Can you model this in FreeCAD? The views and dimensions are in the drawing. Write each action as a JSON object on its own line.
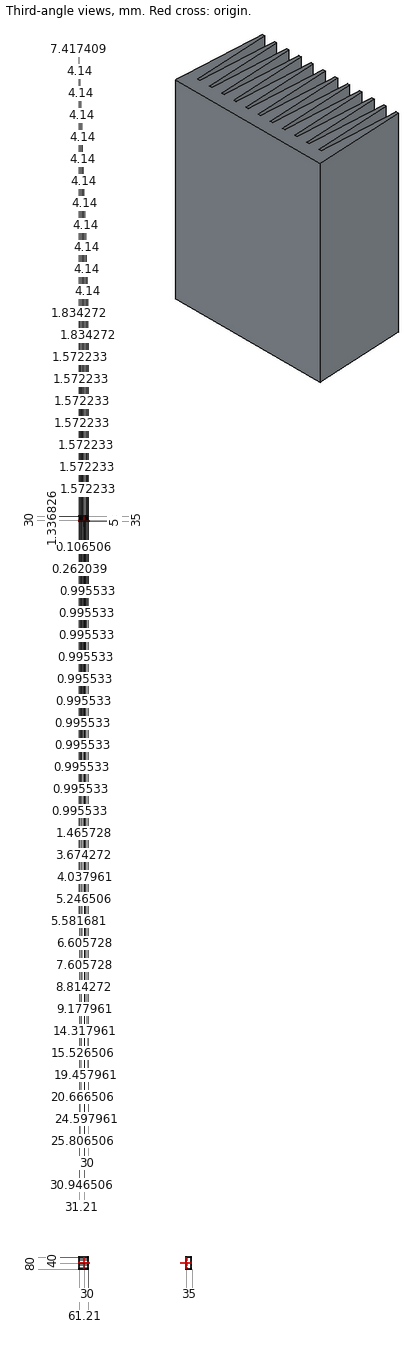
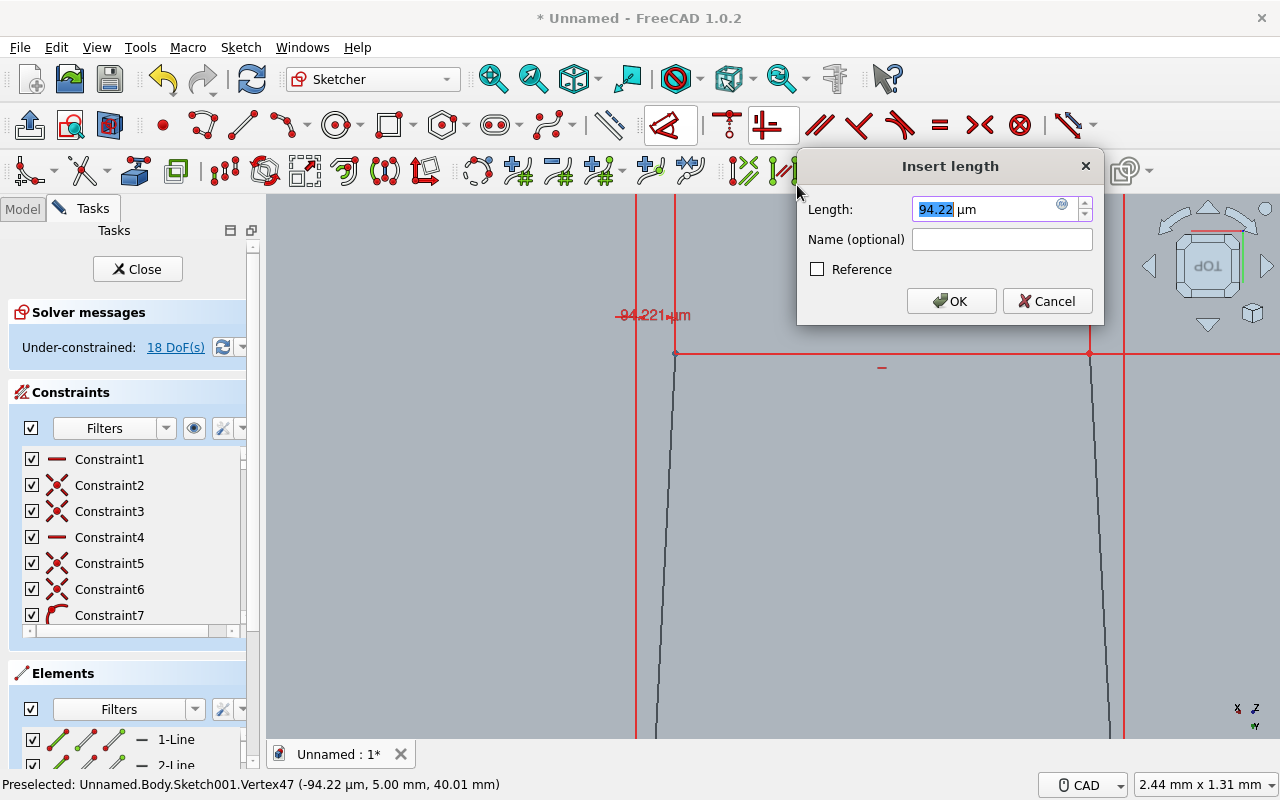
{"action": "key", "text": "ctrl+a"}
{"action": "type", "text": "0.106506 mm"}
{"action": "key", "text": "Return"}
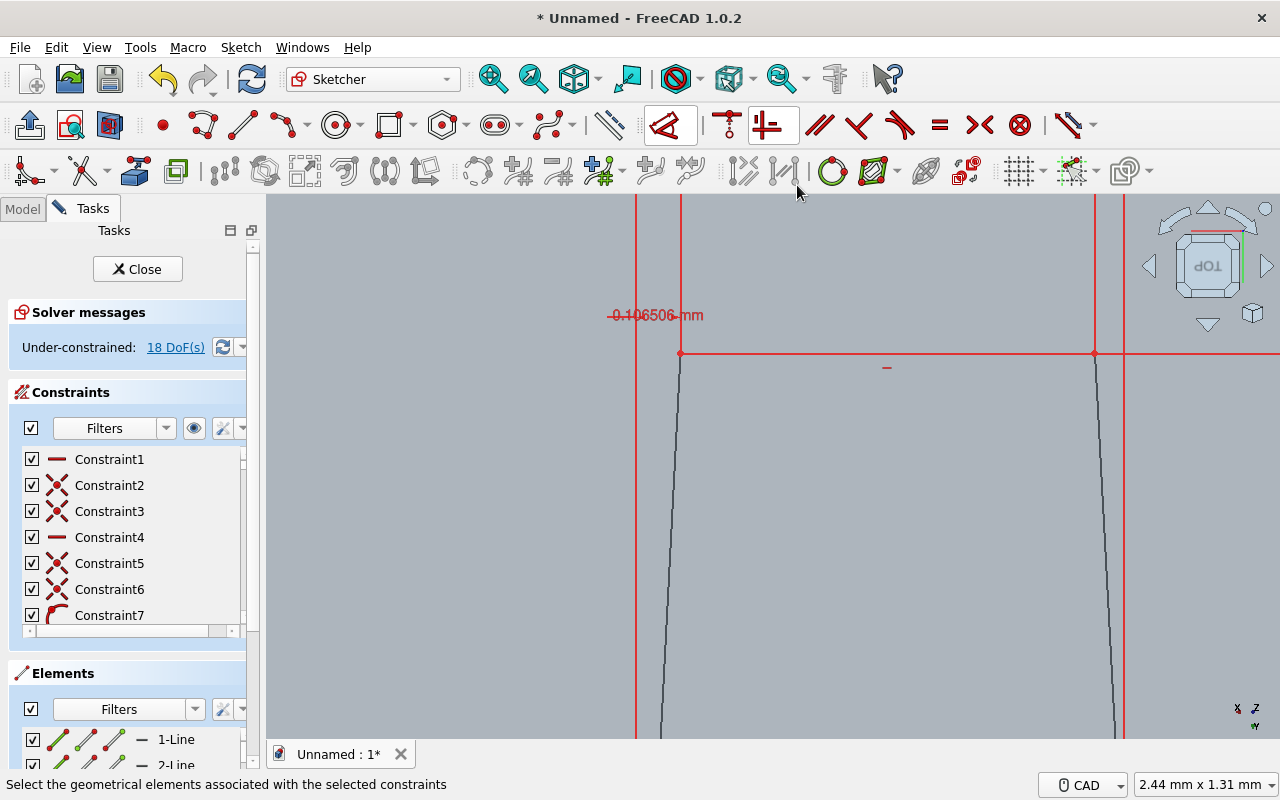
{"action": "scroll", "coordinate": [699, 323], "scroll_direction": "down", "scroll_amount": 18}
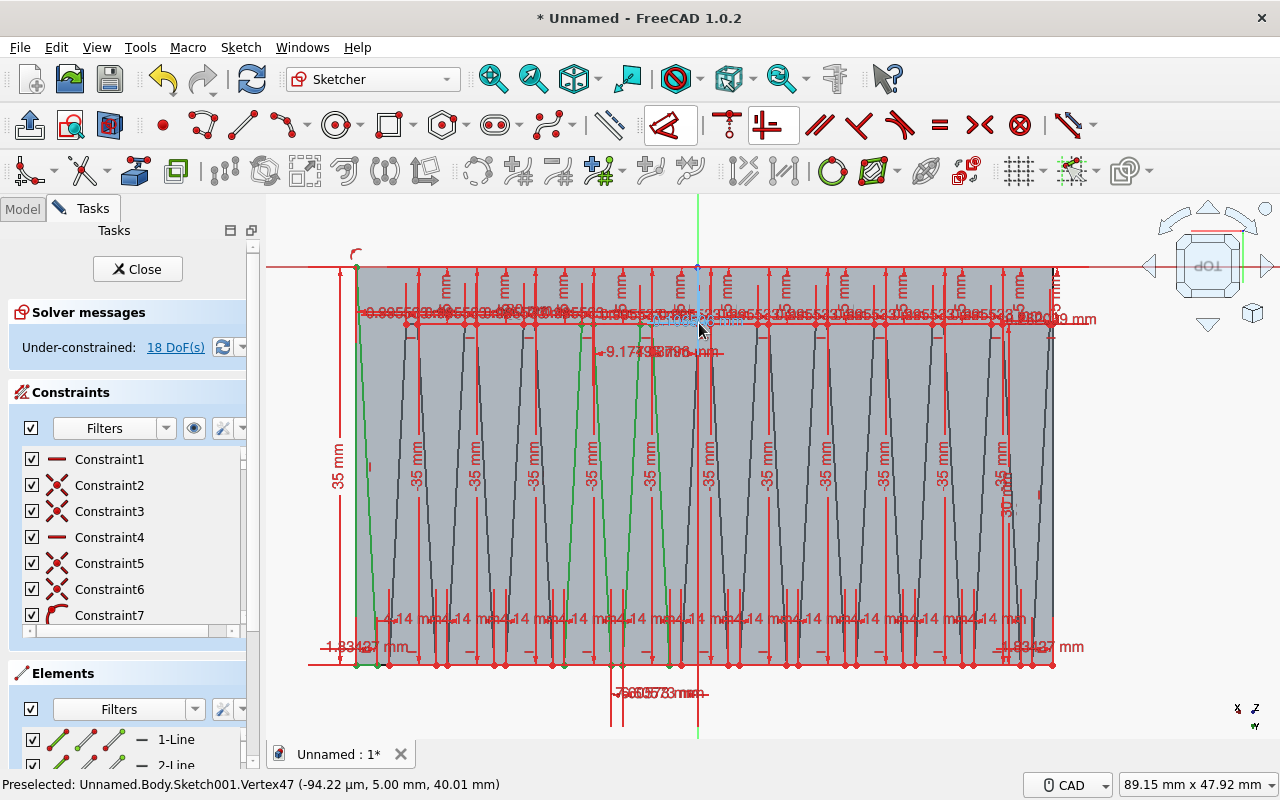
{"action": "scroll", "coordinate": [681, 665], "scroll_direction": "up", "scroll_amount": 5}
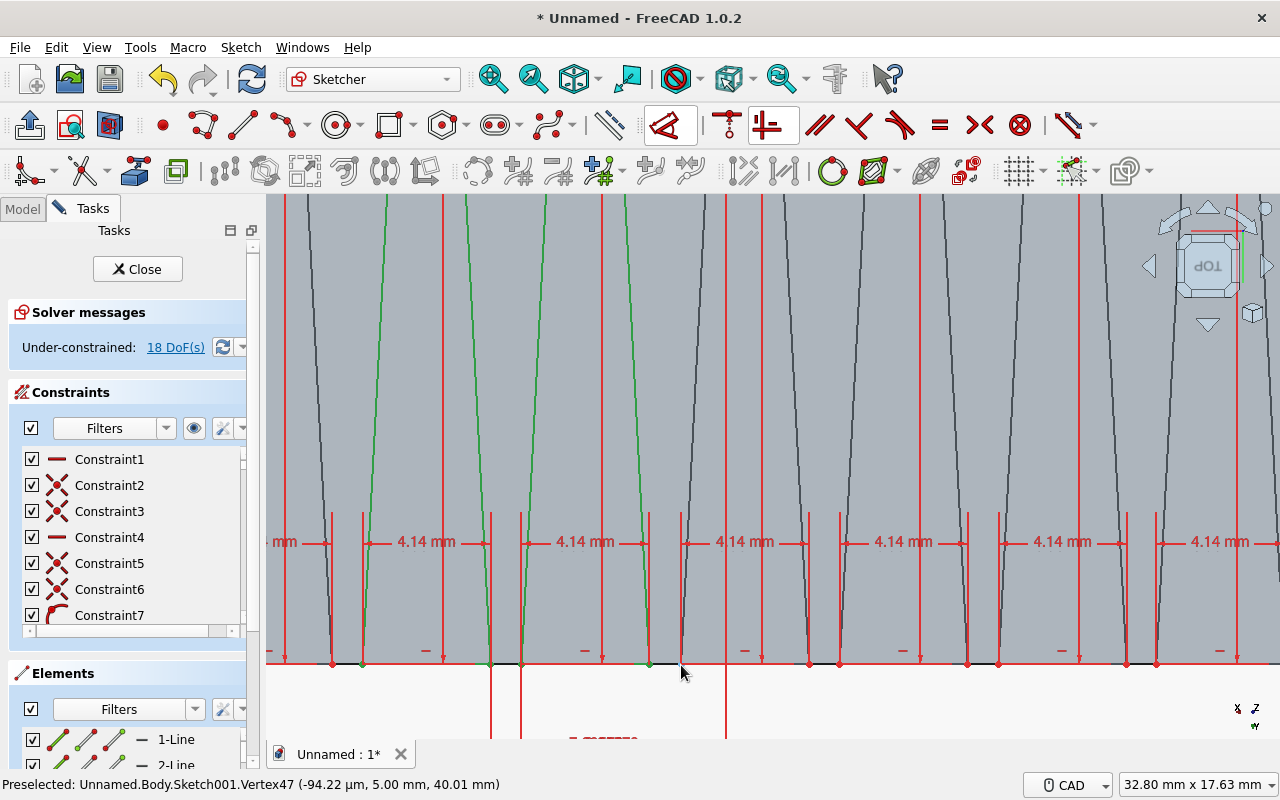
{"action": "left_click", "coordinate": [681, 664]}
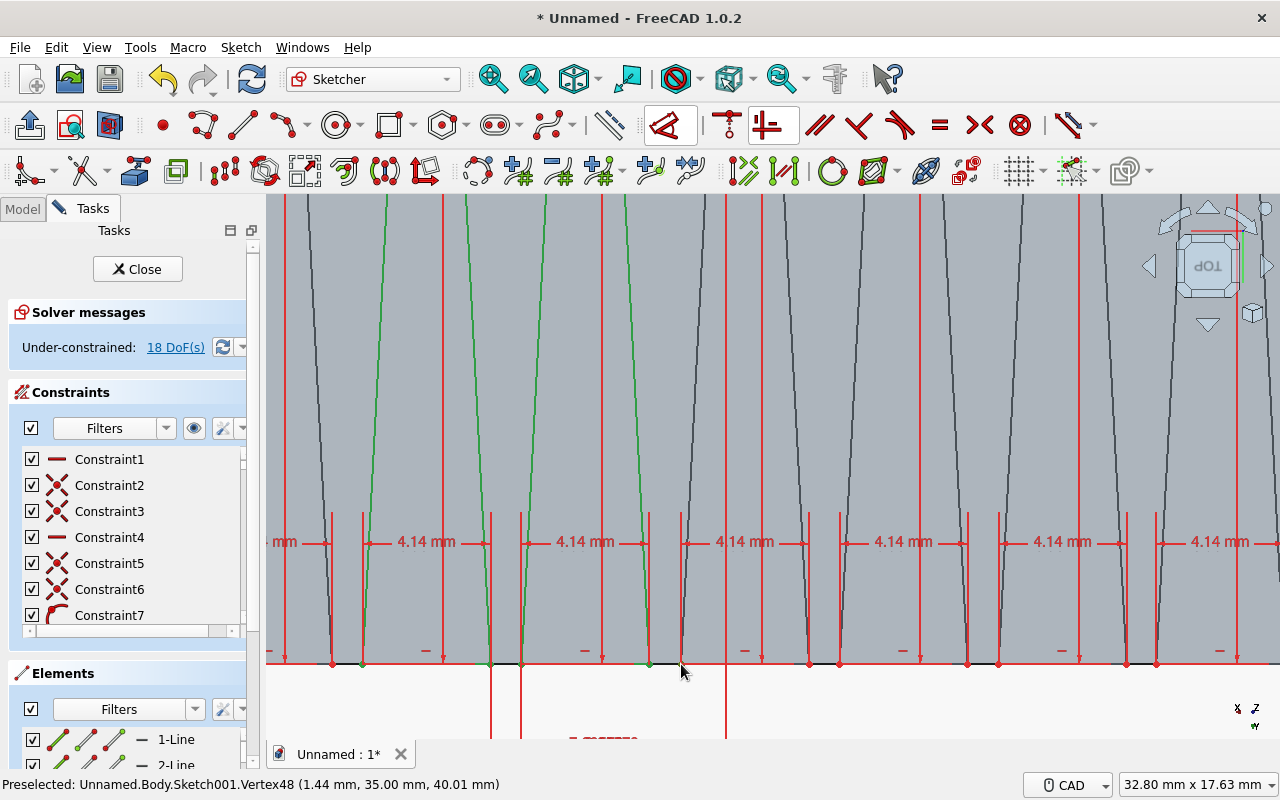
{"action": "key", "text": "l"}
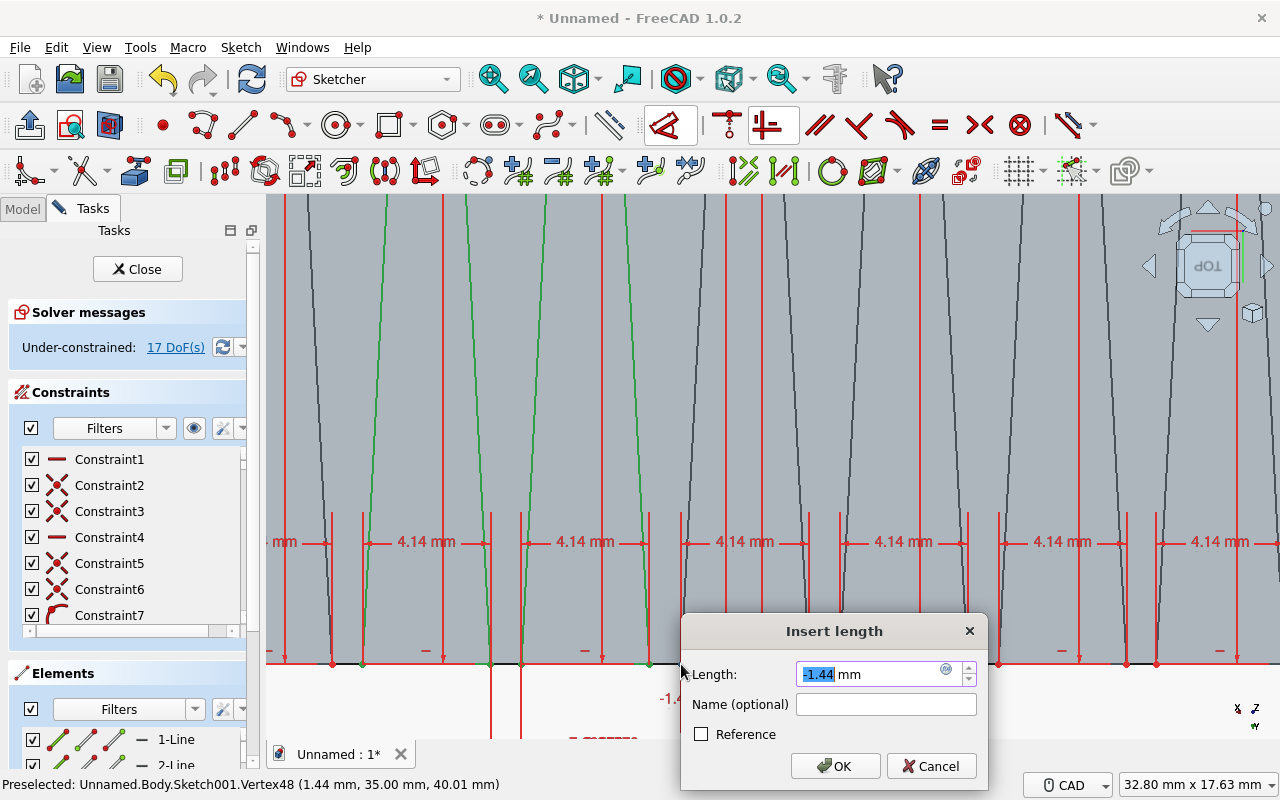
{"action": "type", "text": "-1.465728"}
{"action": "key", "text": "Return"}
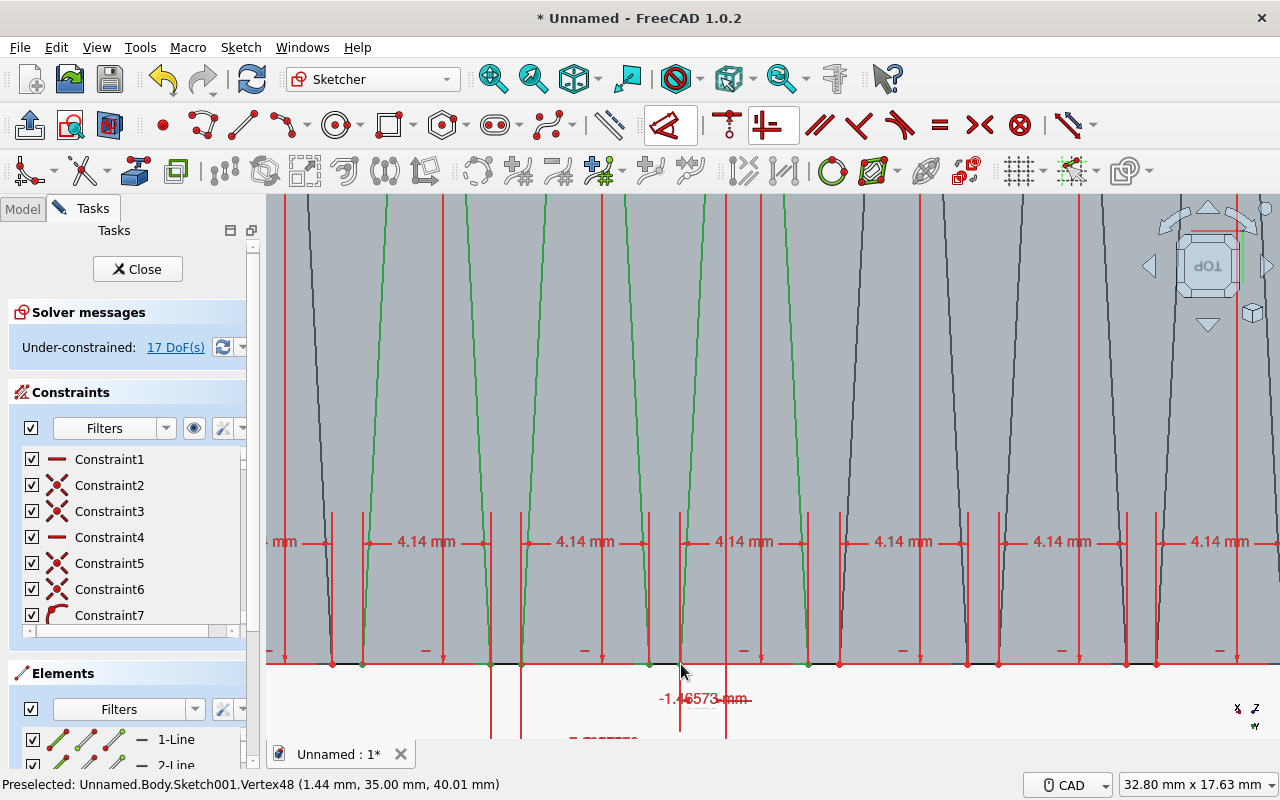
{"action": "scroll", "coordinate": [687, 614], "scroll_direction": "down", "scroll_amount": 6}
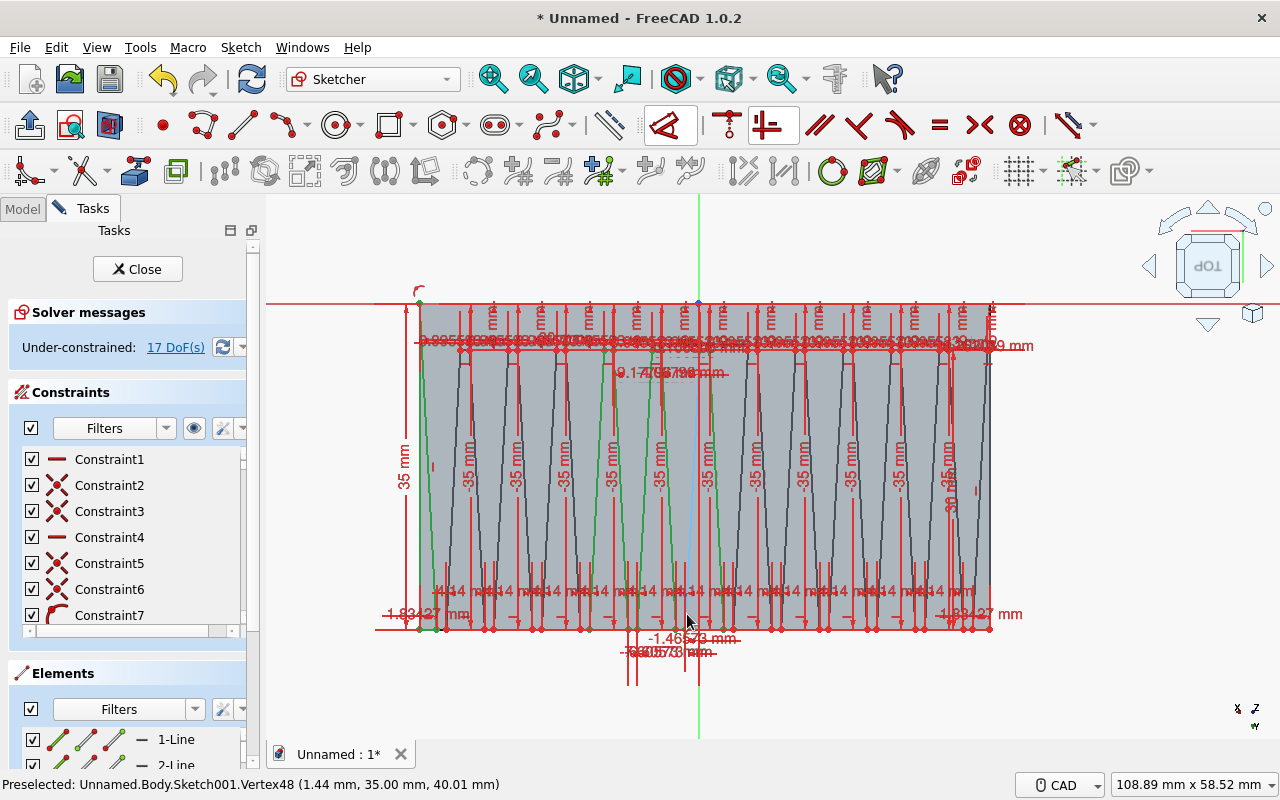
{"action": "scroll", "coordinate": [748, 350], "scroll_direction": "up", "scroll_amount": 2}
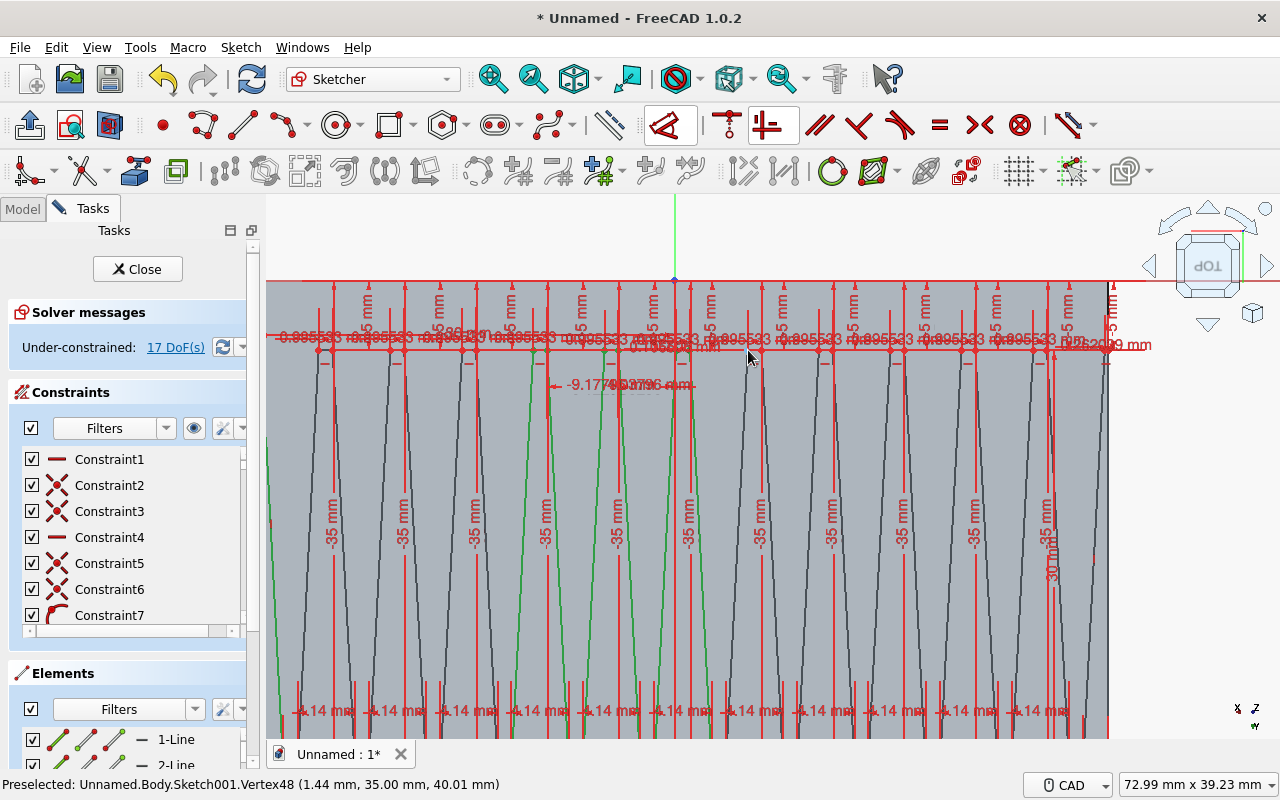
{"action": "left_click", "coordinate": [748, 350]}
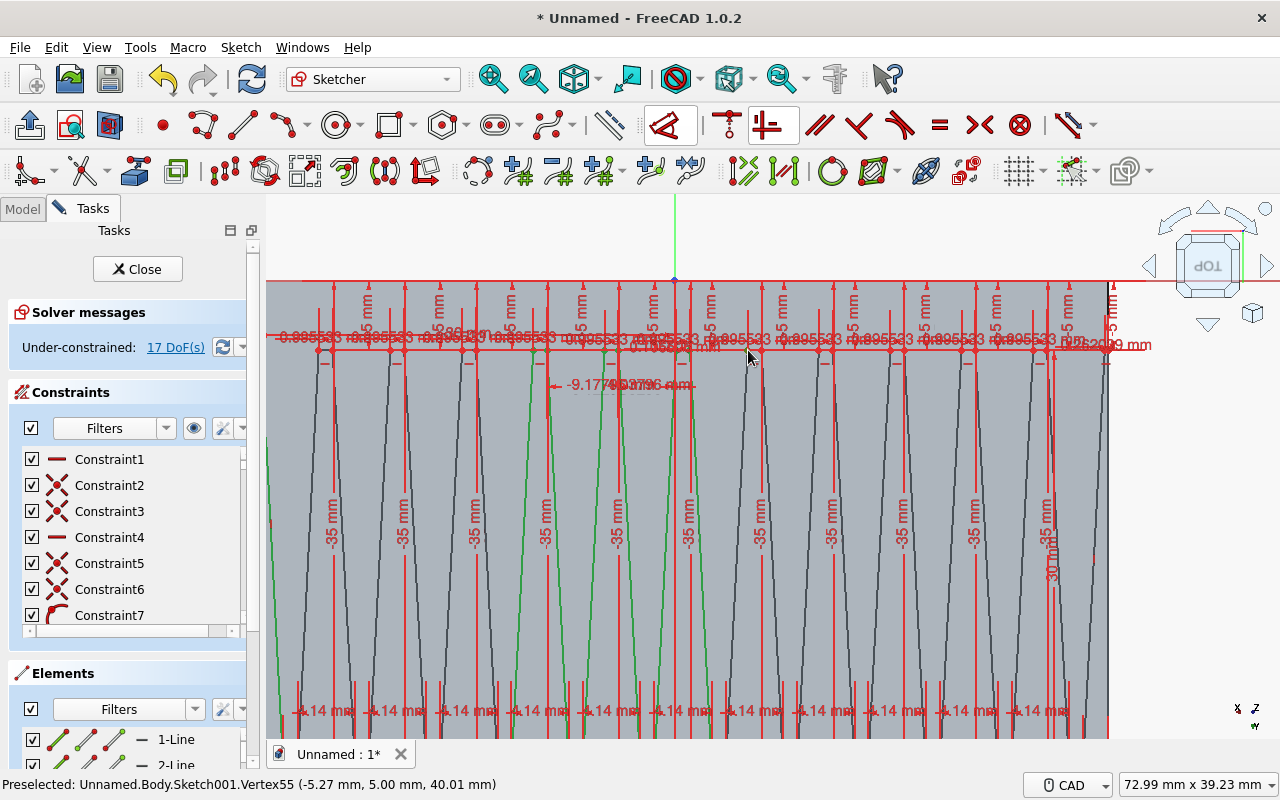
{"action": "left_click", "coordinate": [692, 126]}